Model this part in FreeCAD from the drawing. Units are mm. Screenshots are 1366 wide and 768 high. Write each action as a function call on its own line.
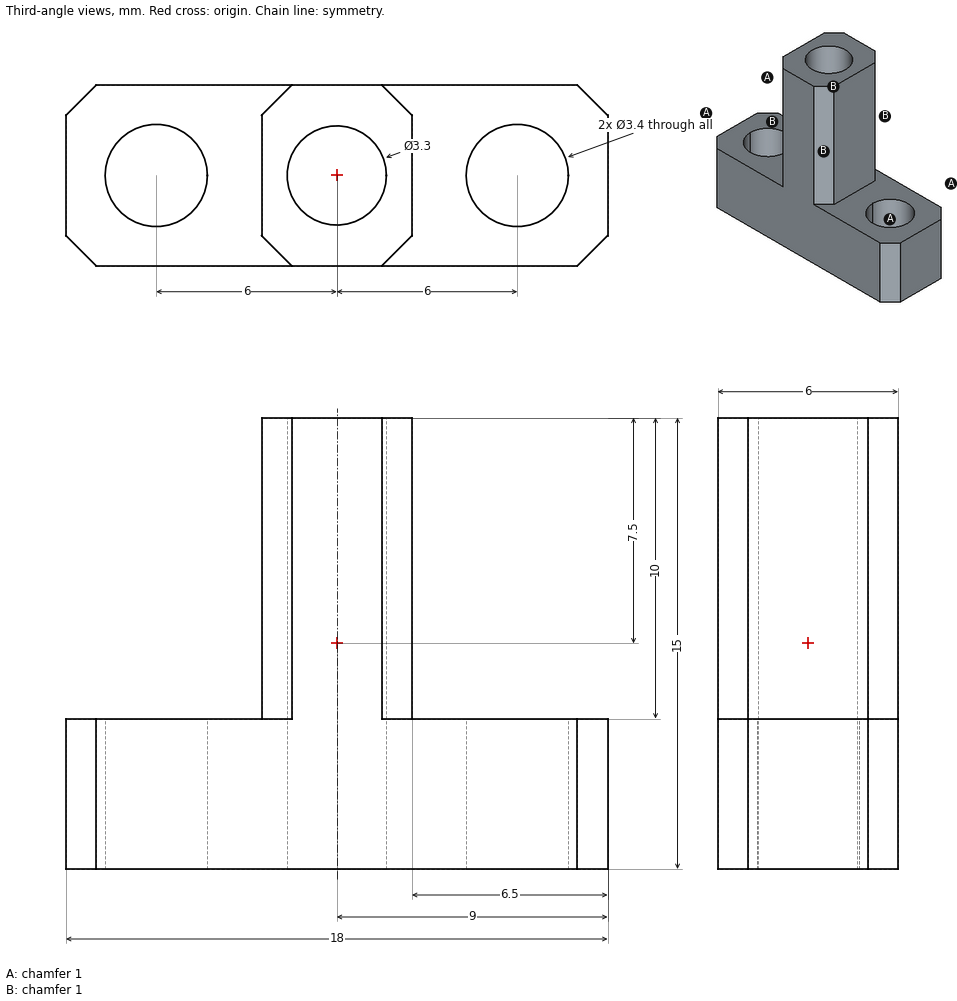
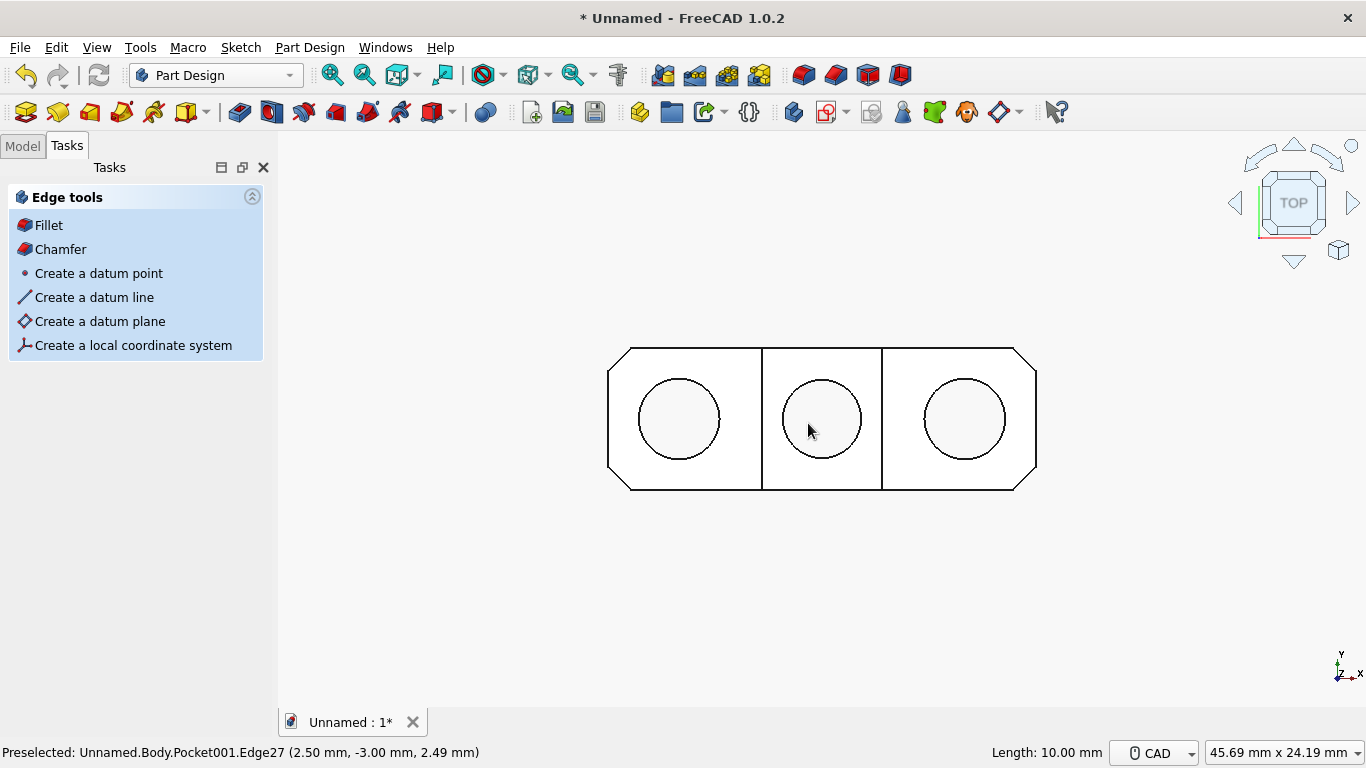
click(334, 76)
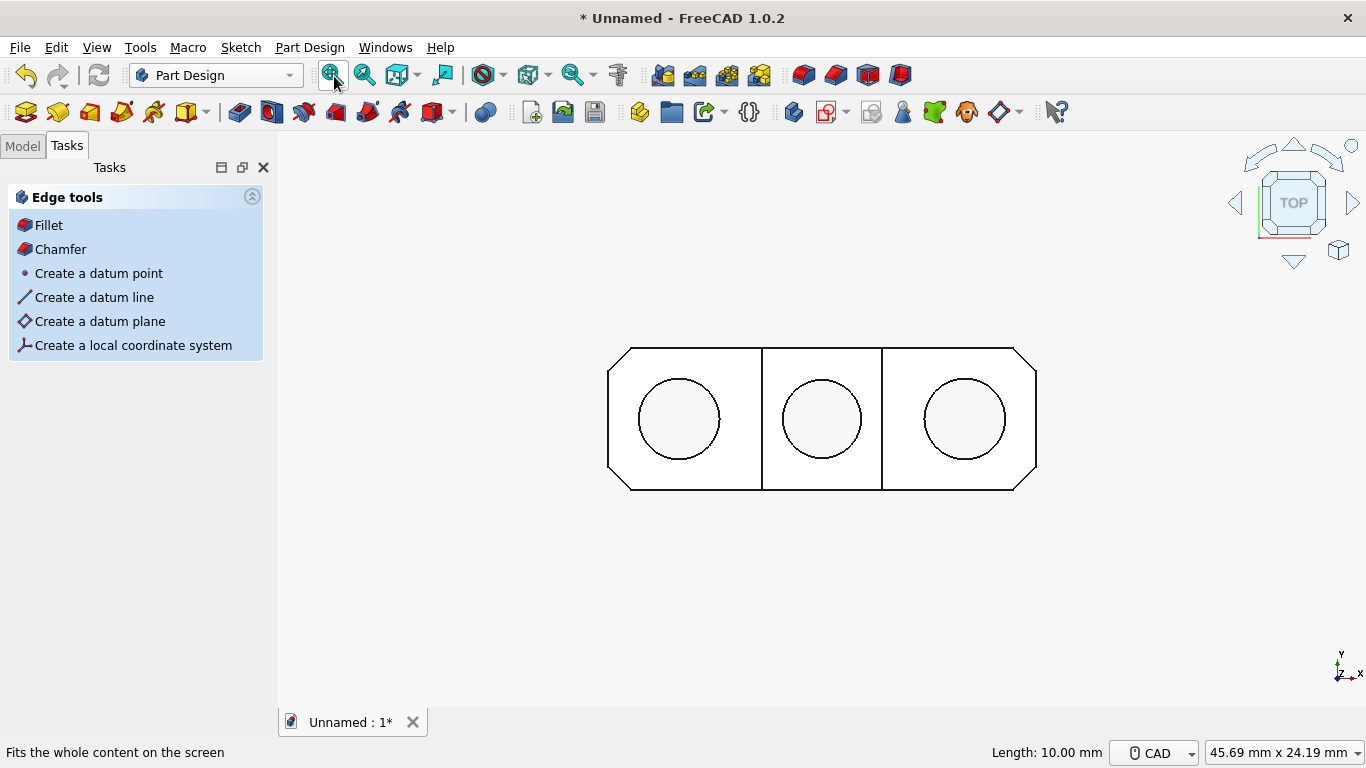
key(1)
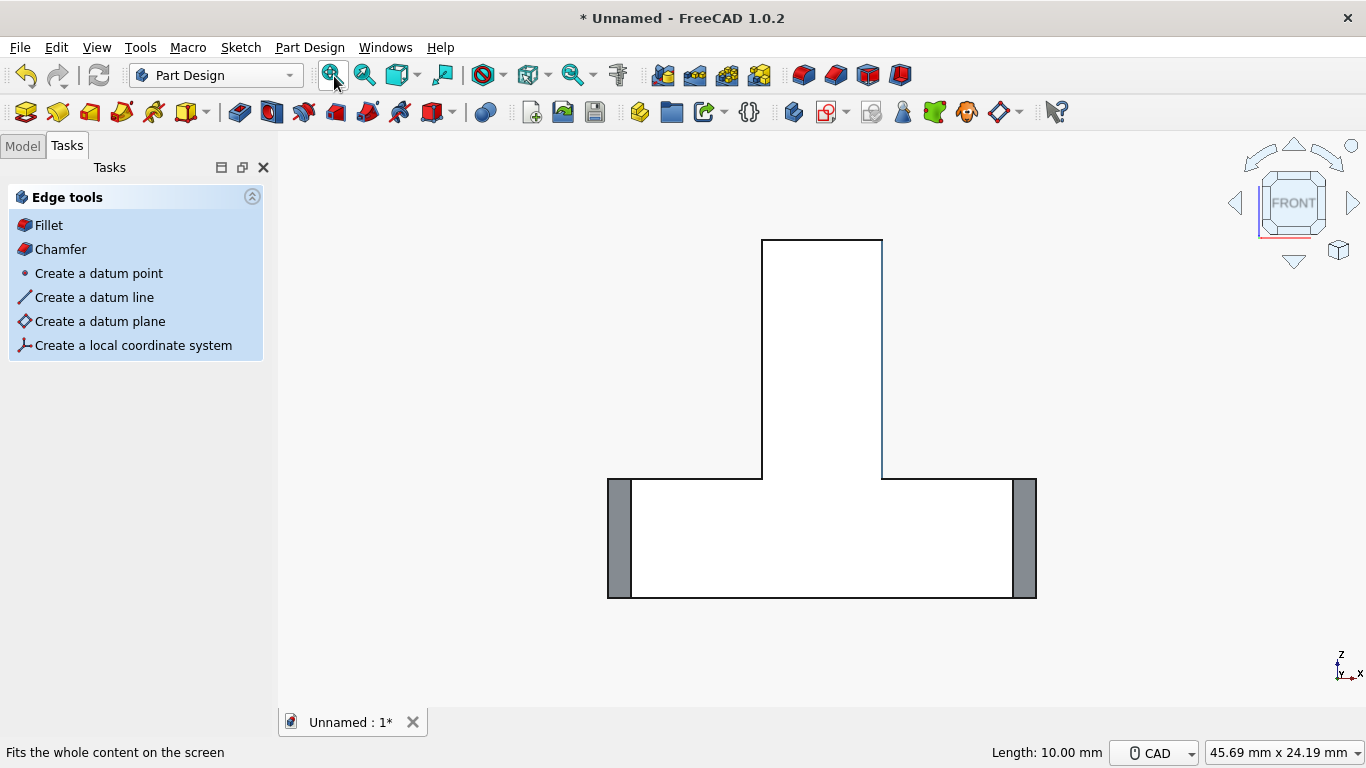
click(762, 358, ctrl)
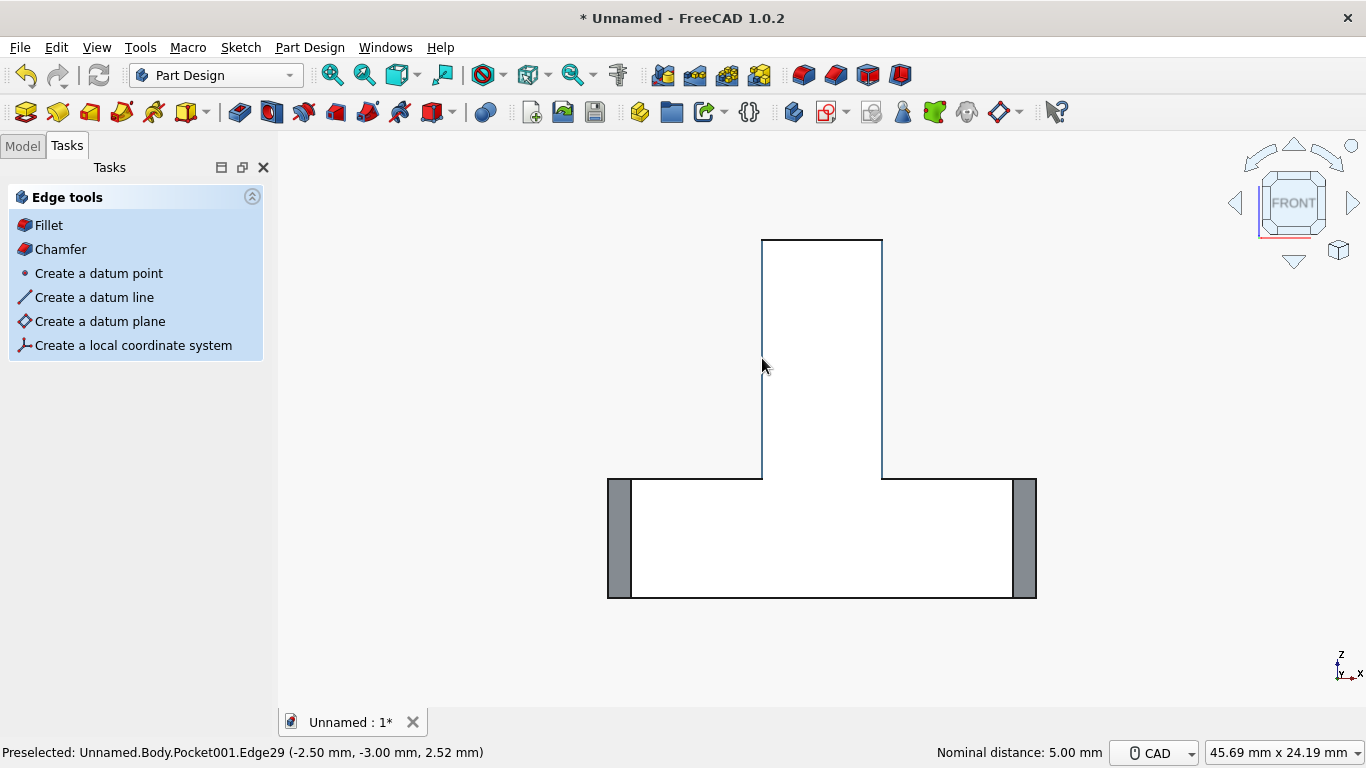
key(3)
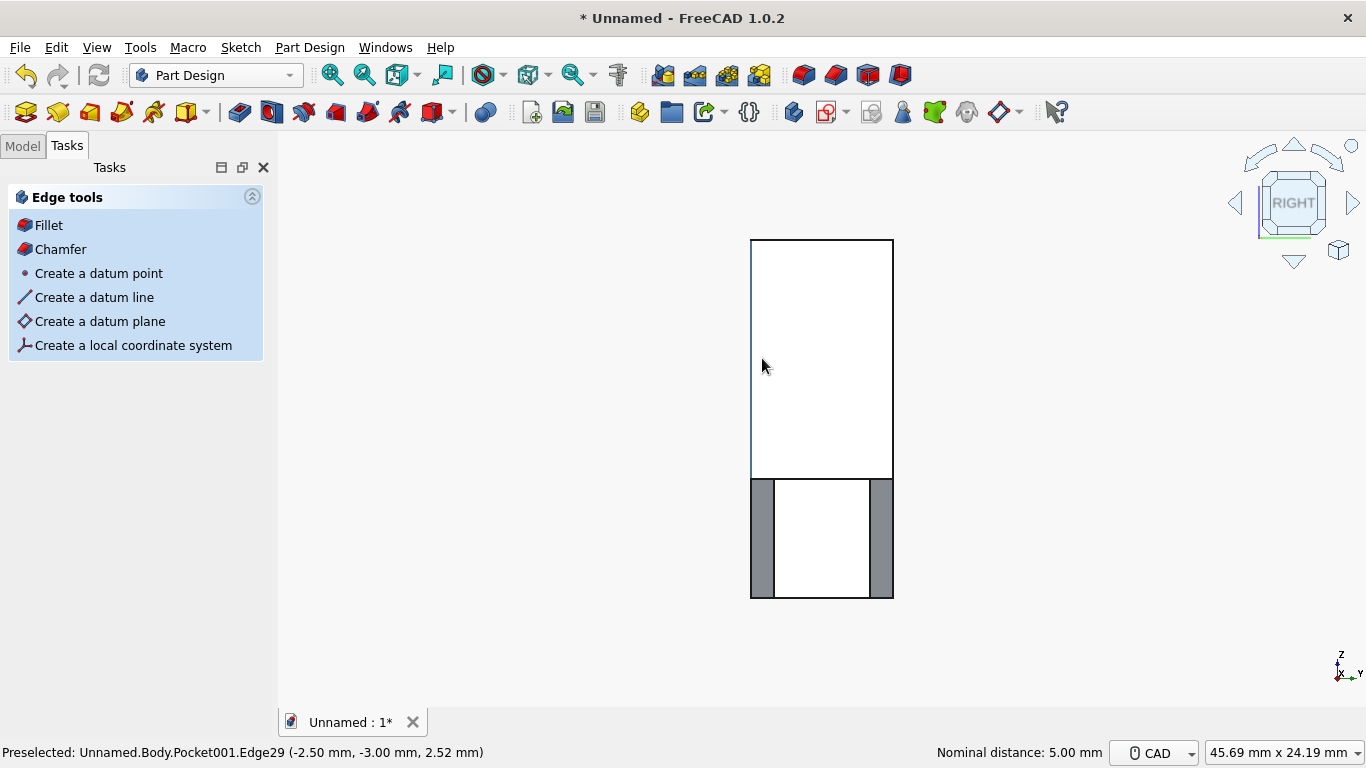
click(893, 358, ctrl)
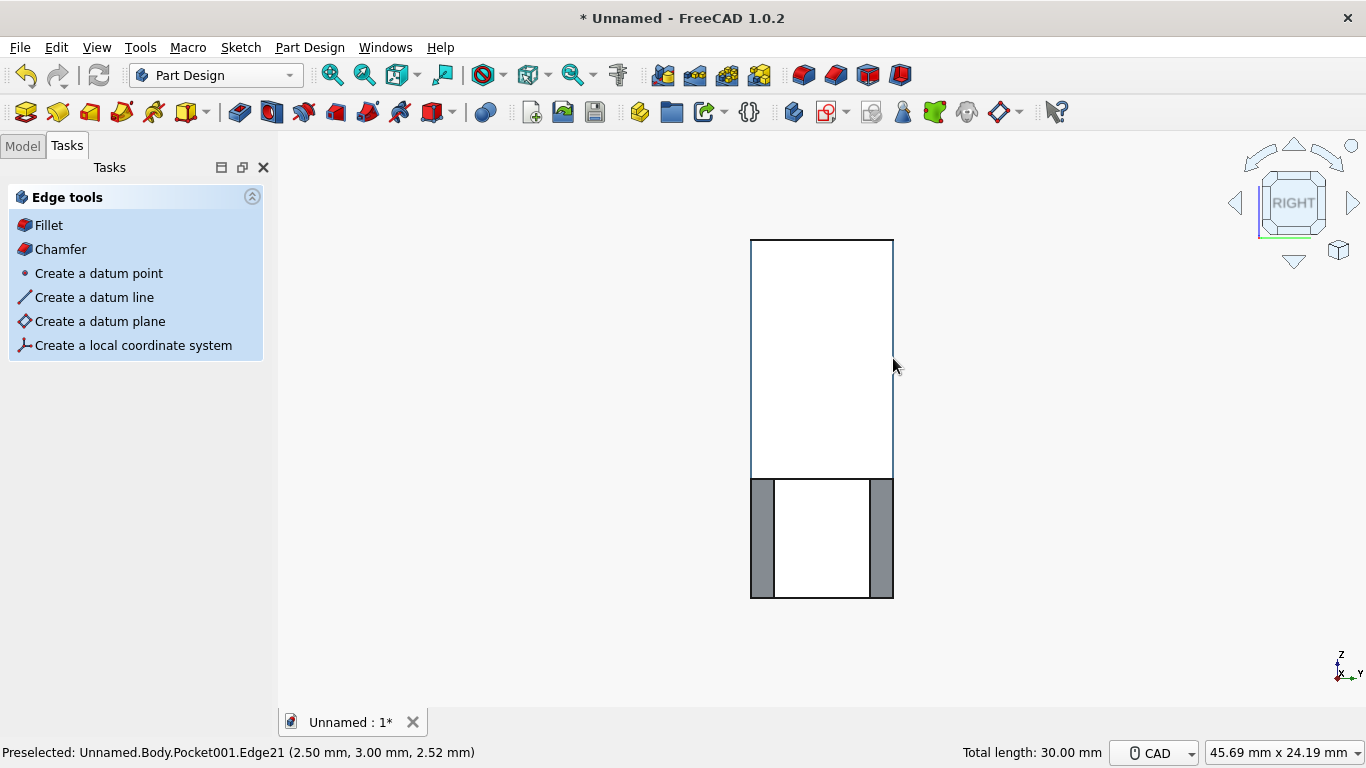
key(5)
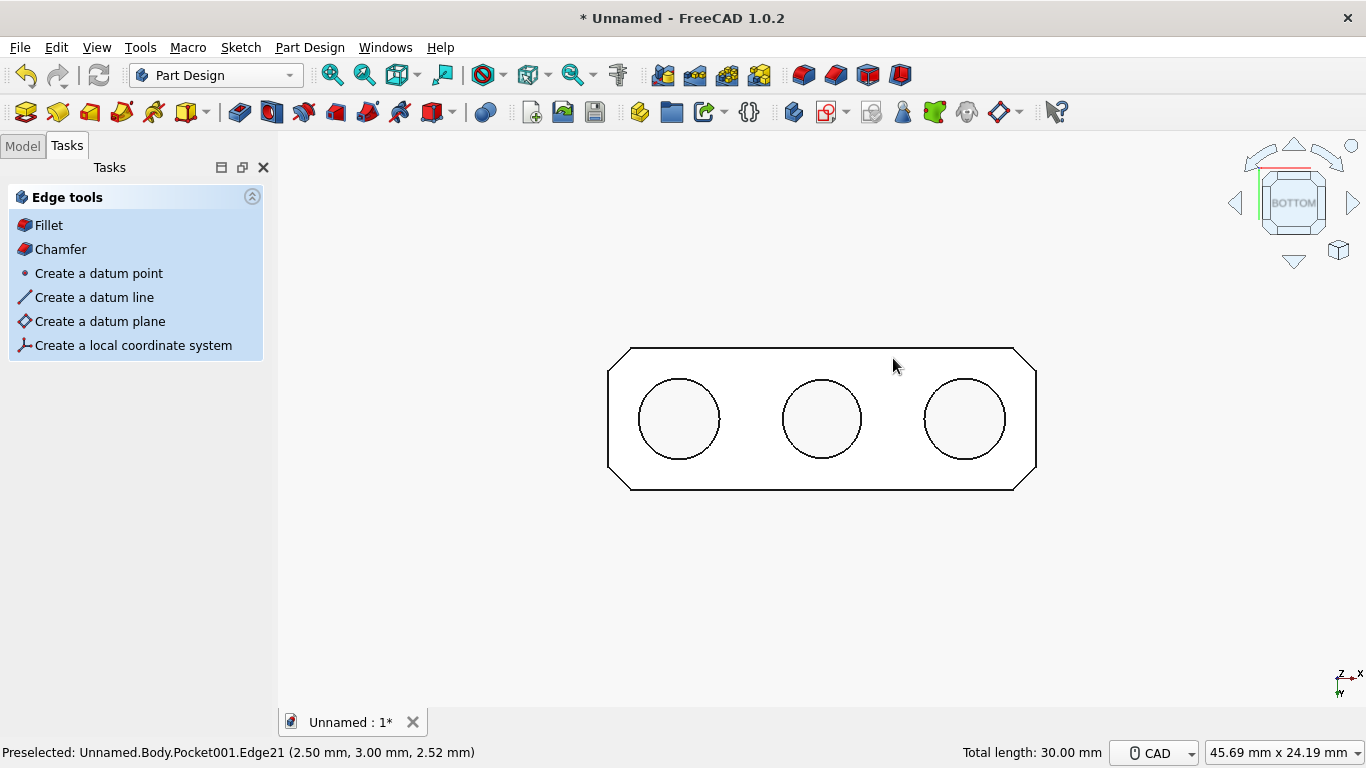
click(334, 76)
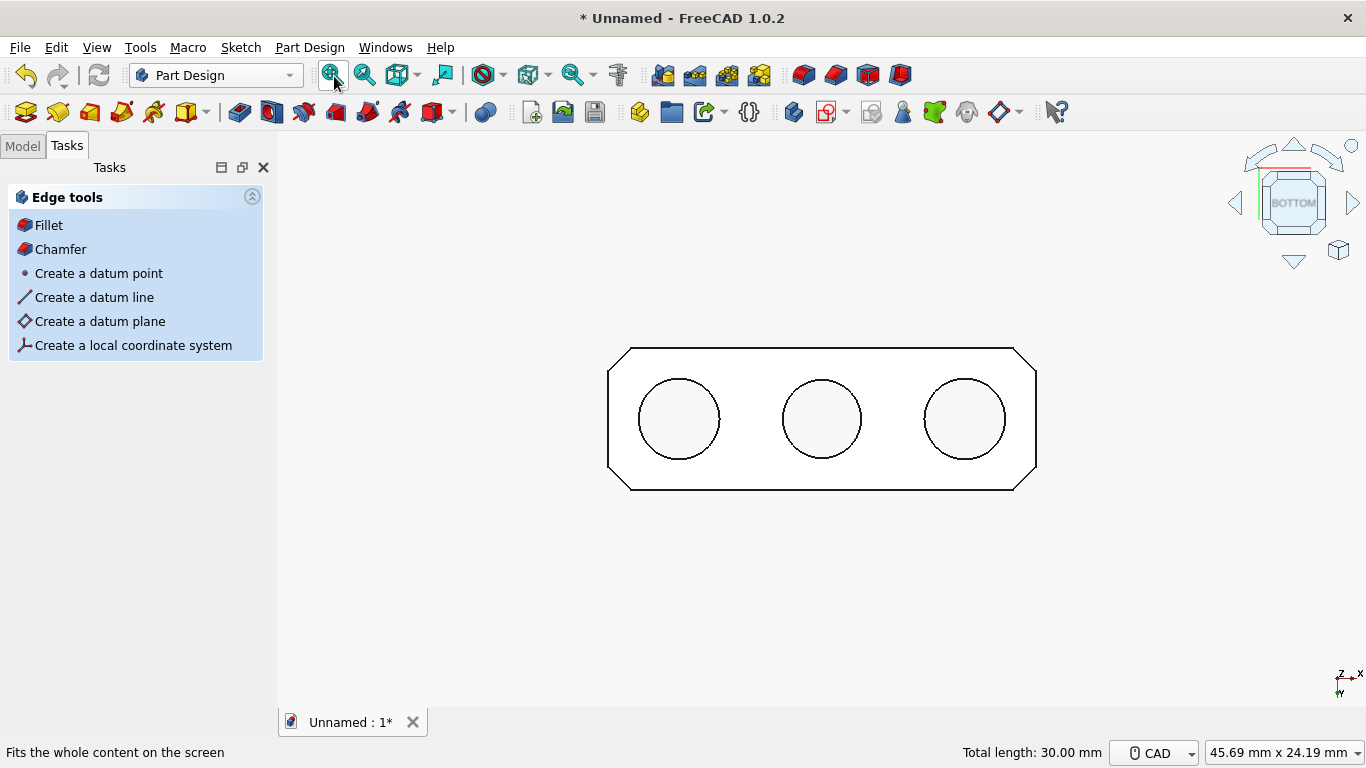
key(4)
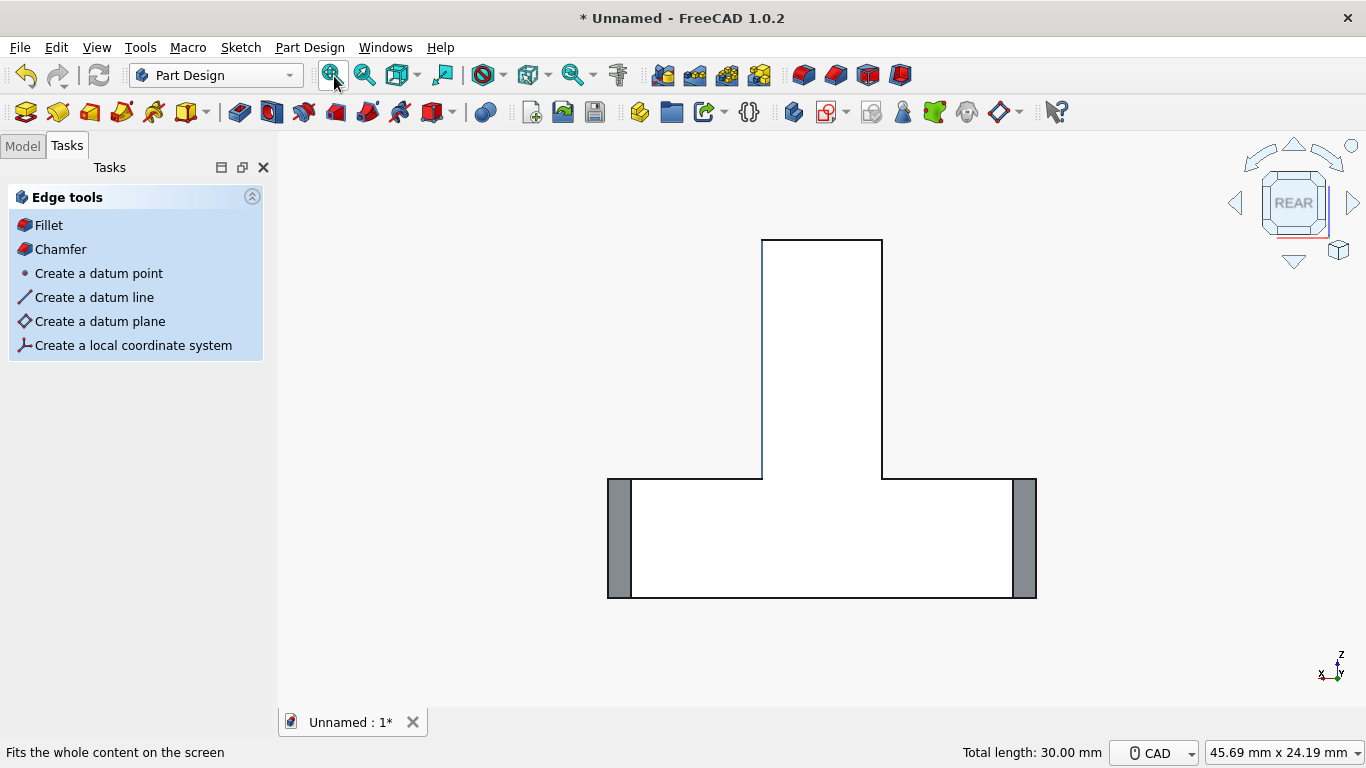
click(882, 358, ctrl)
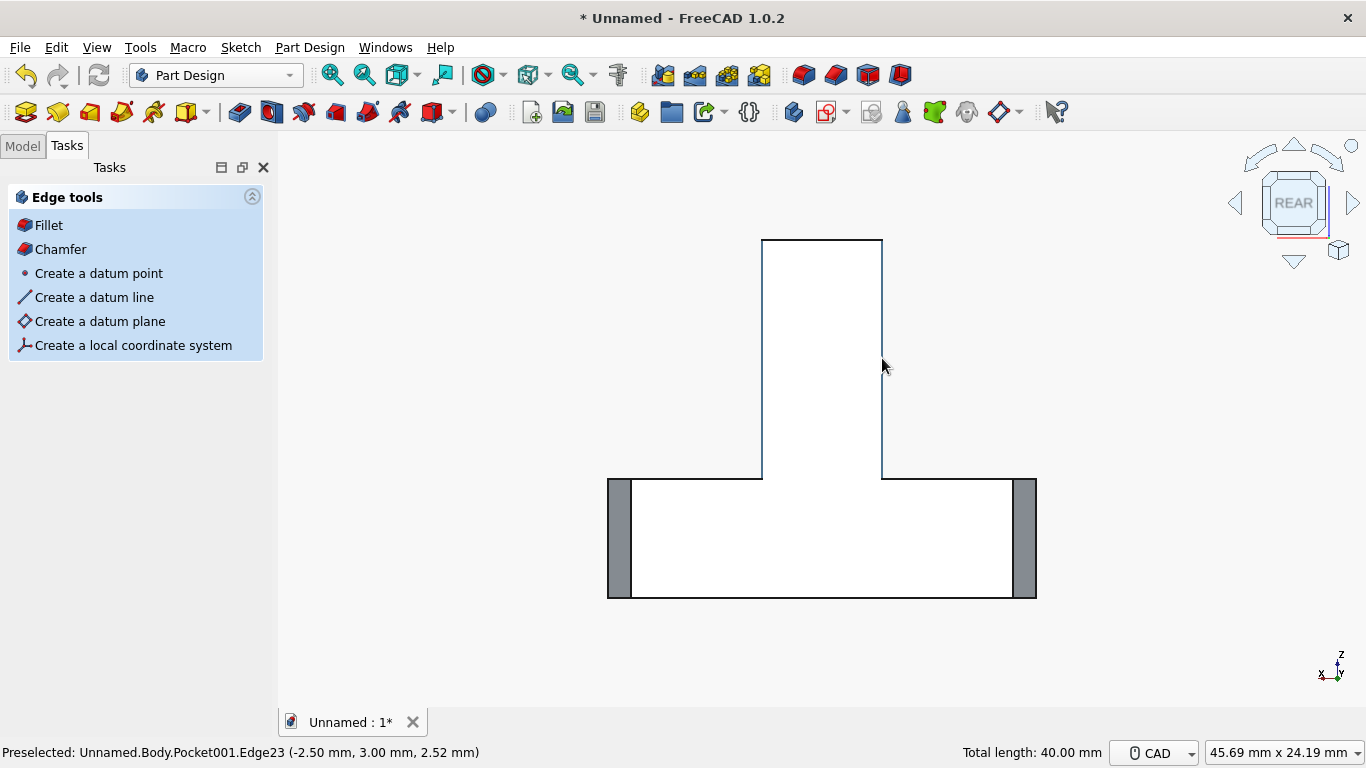
click(836, 76)